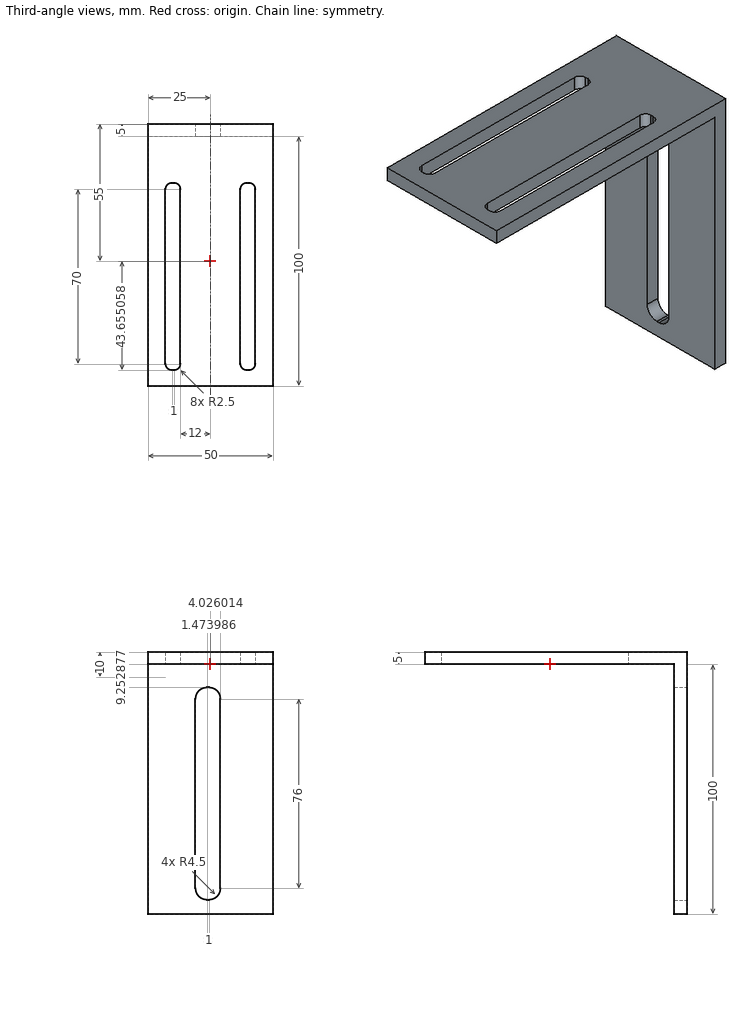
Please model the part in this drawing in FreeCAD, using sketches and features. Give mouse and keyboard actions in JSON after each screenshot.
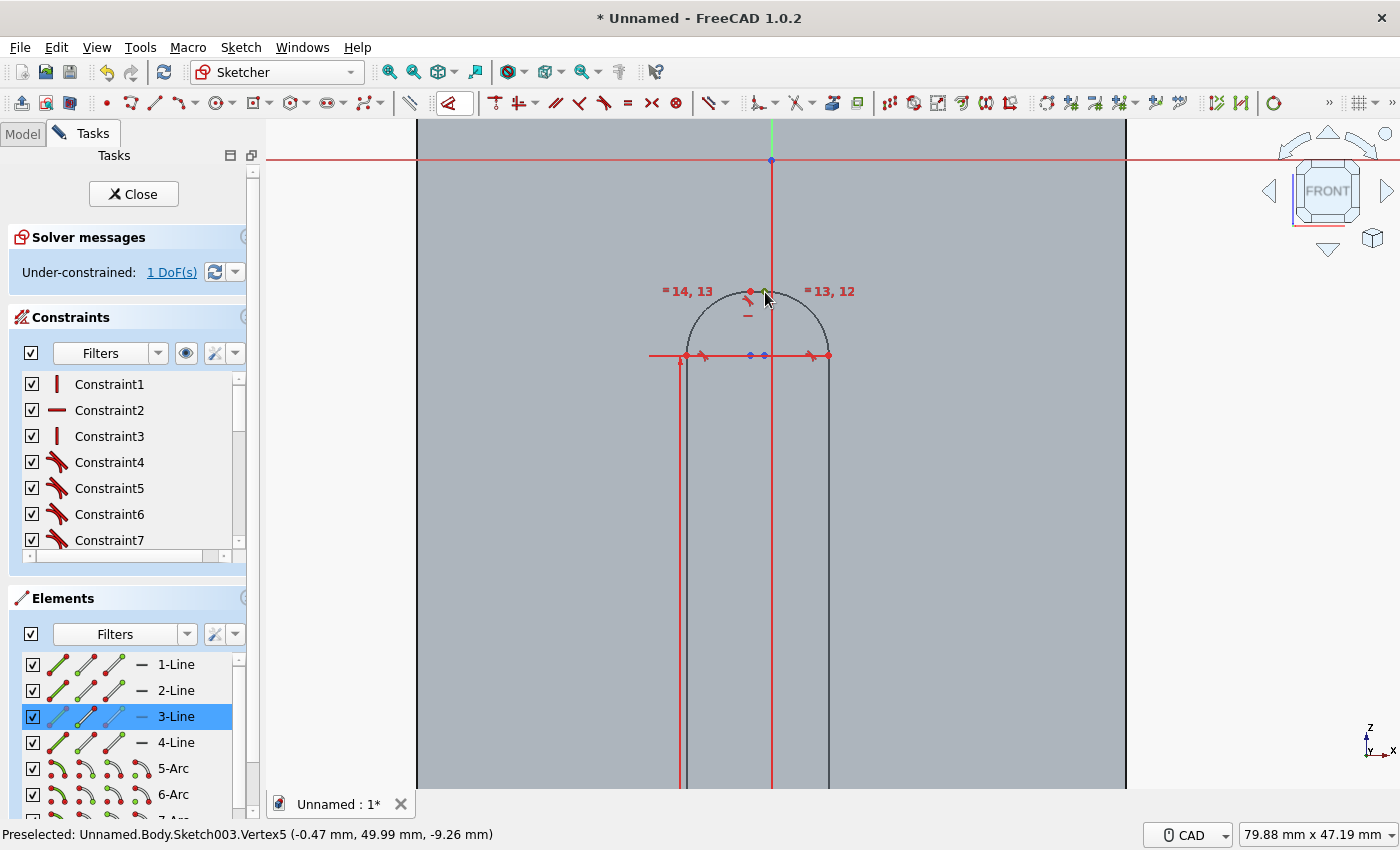
{"action": "key", "text": "i"}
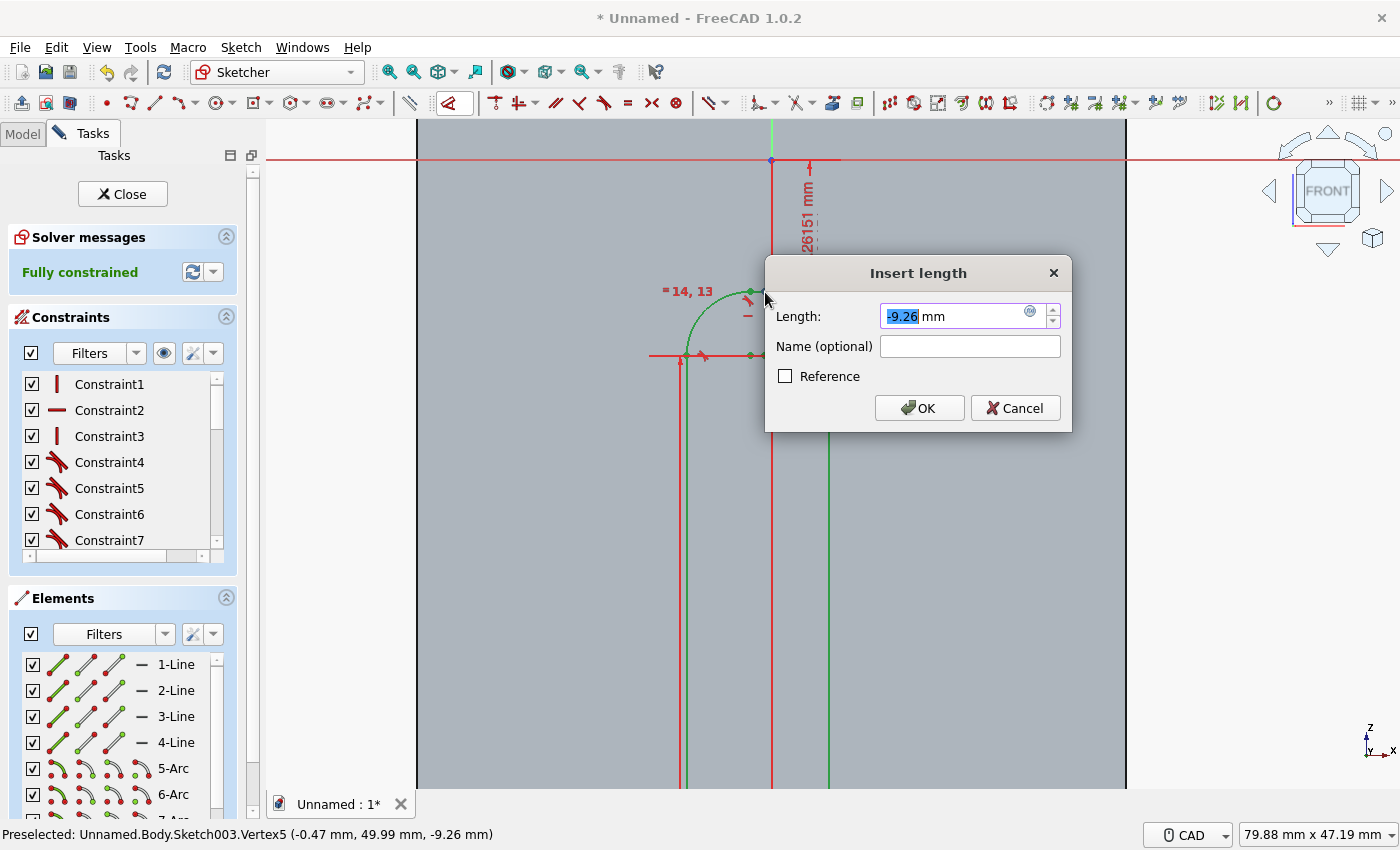
{"action": "type", "text": "-9.252877"}
{"action": "key", "text": "Return"}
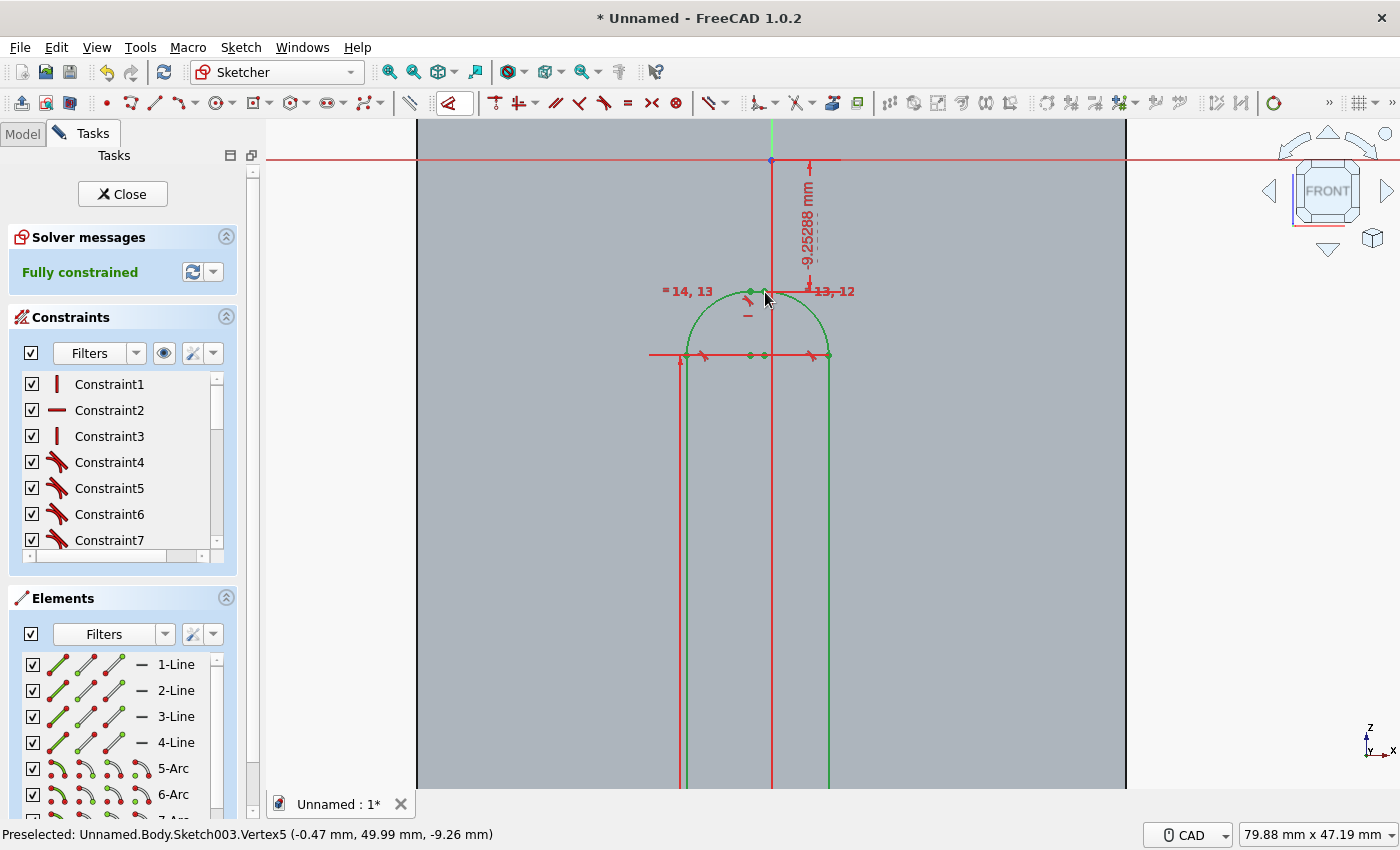
{"action": "left_click", "coordinate": [123, 194]}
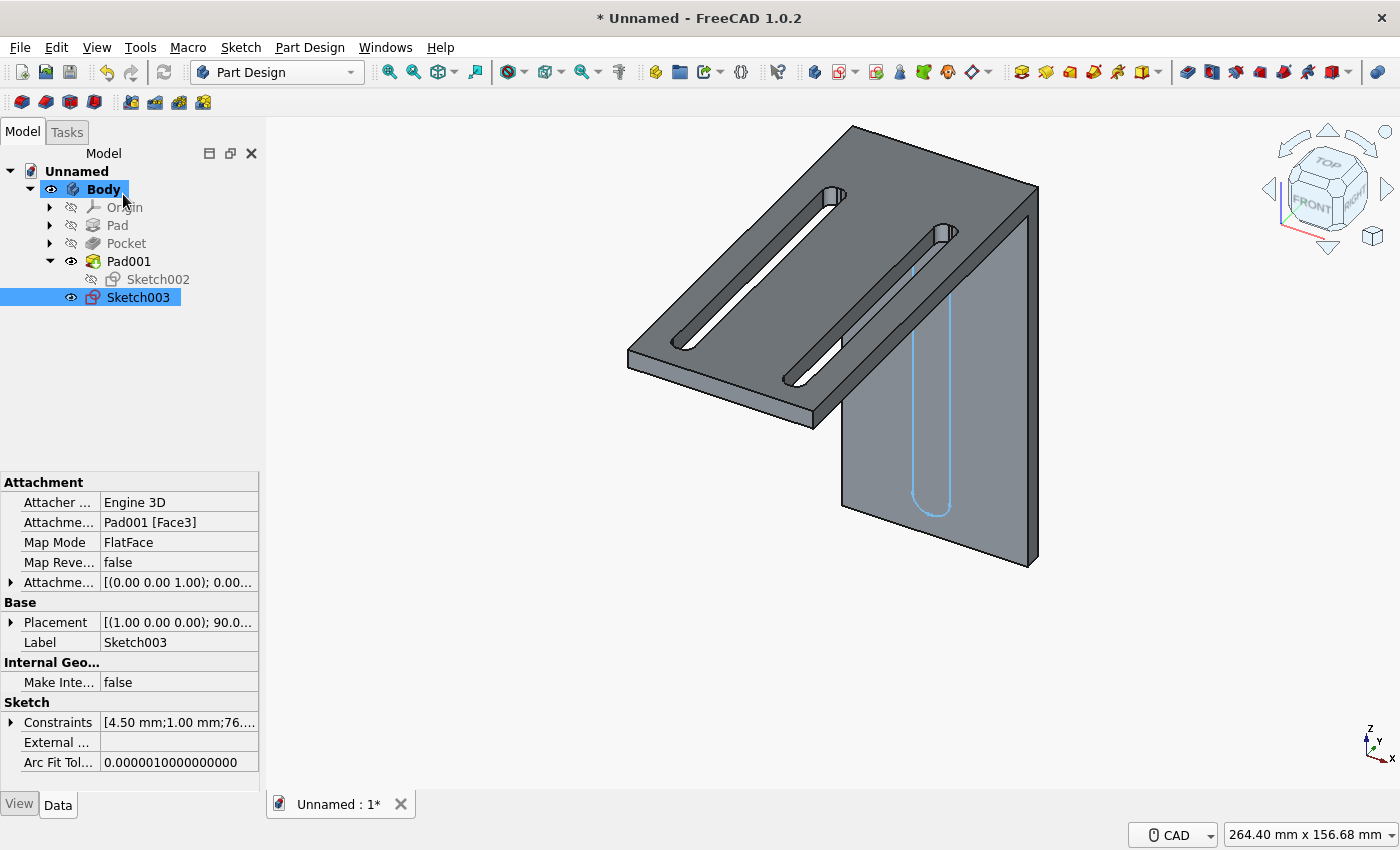
{"action": "left_click", "coordinate": [1188, 72]}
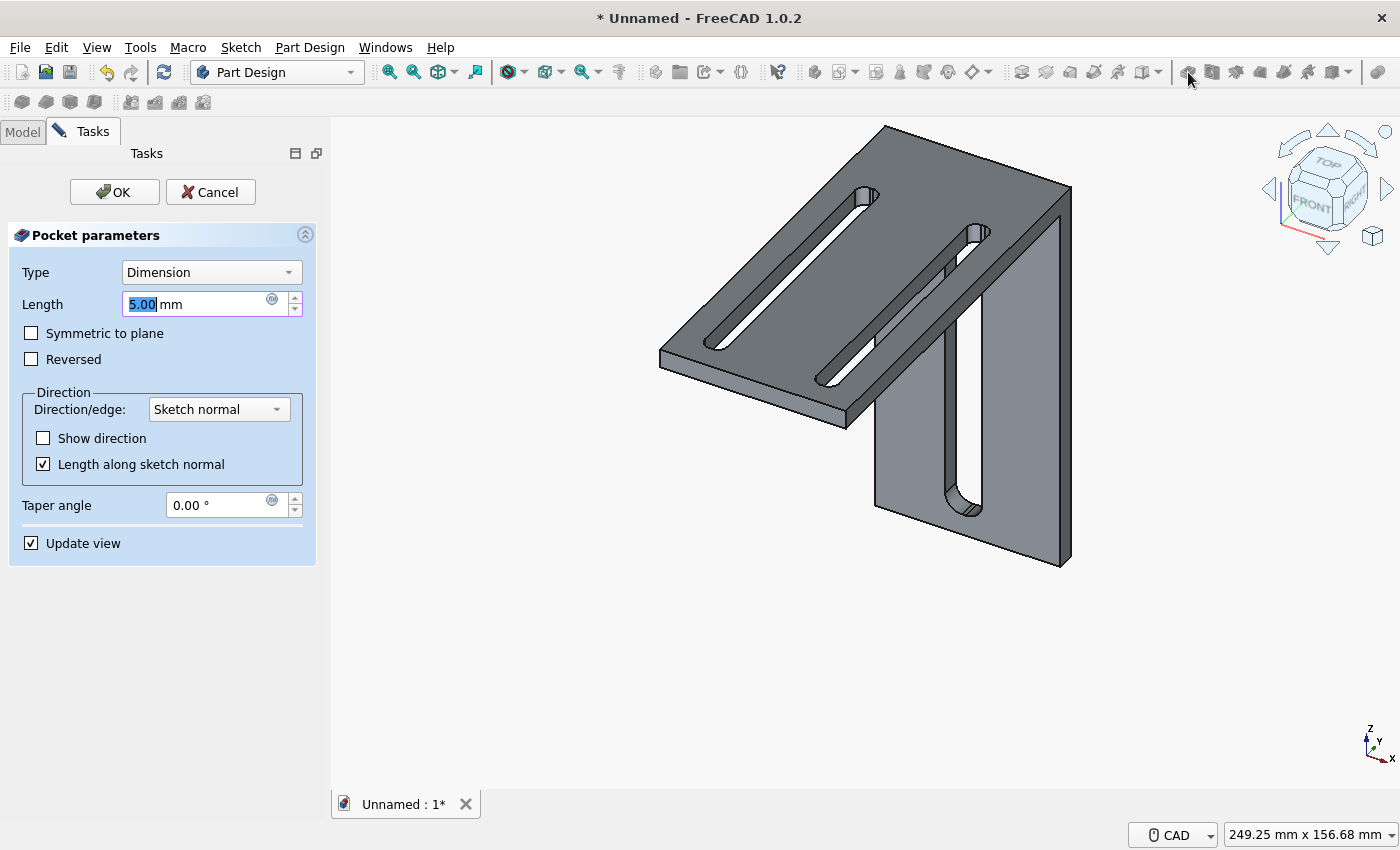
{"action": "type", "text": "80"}
{"action": "key", "text": "Tab"}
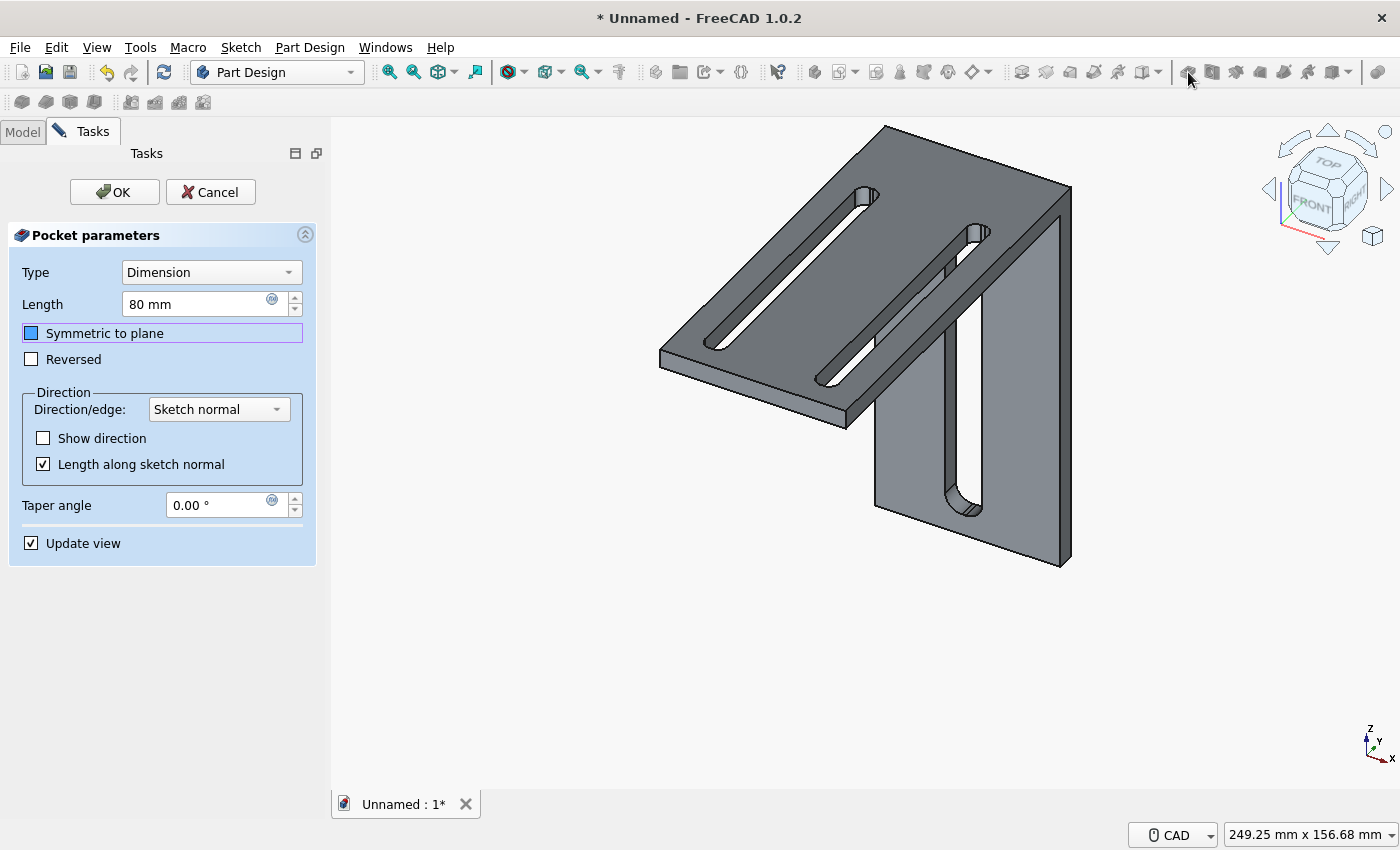
{"action": "left_click", "coordinate": [115, 192]}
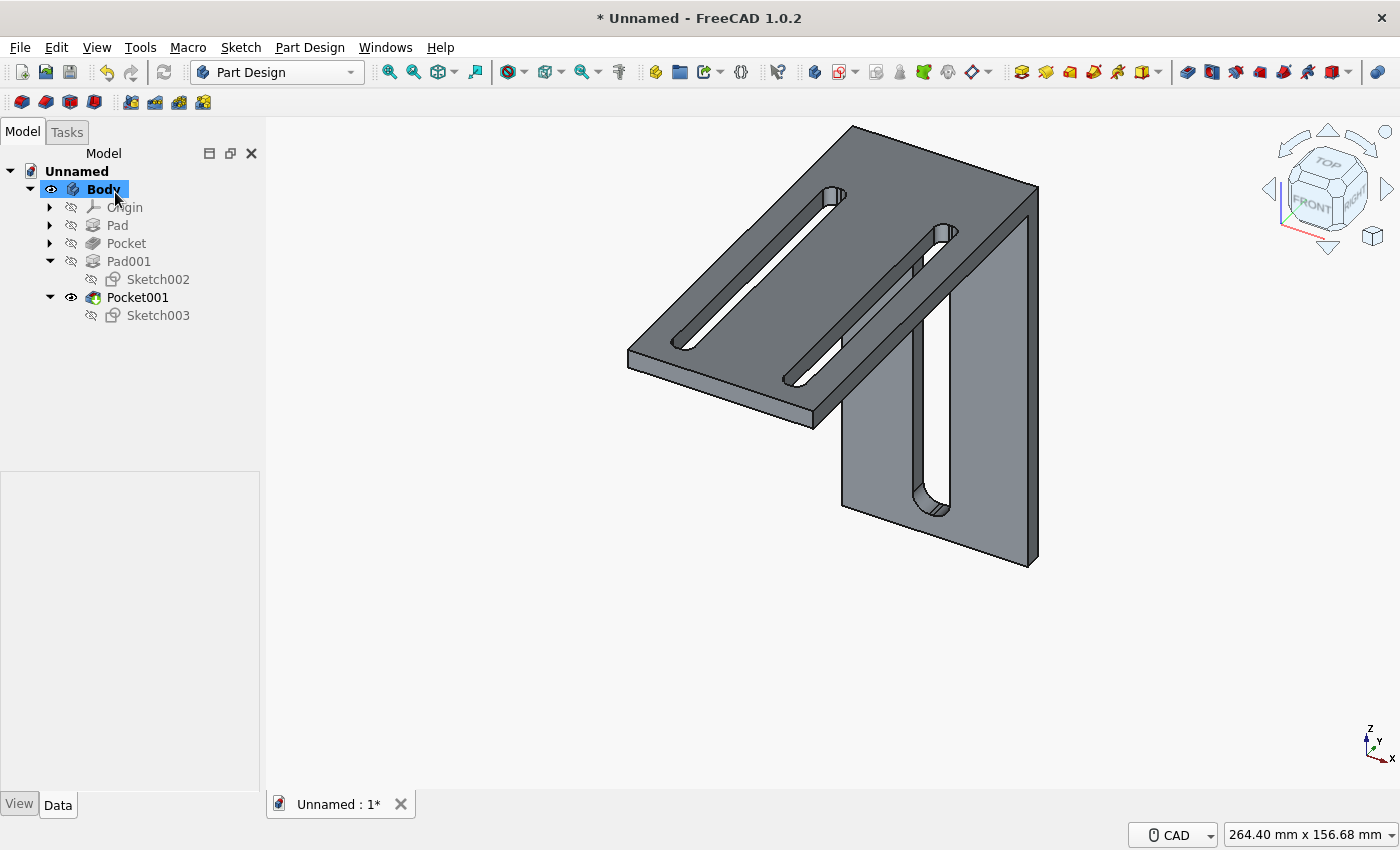
{"action": "key", "text": "0"}